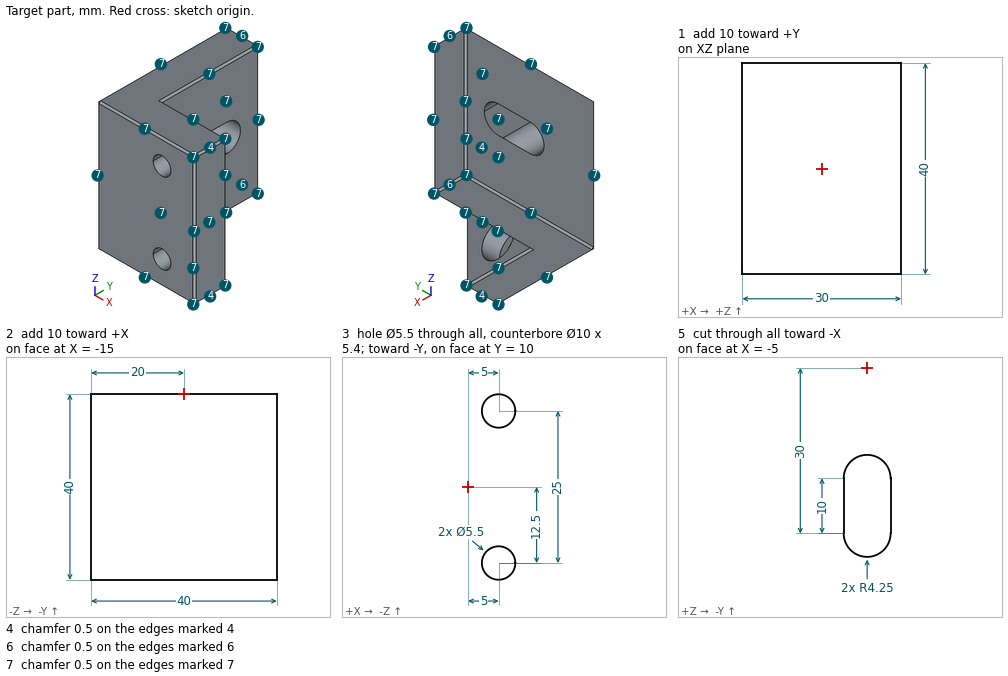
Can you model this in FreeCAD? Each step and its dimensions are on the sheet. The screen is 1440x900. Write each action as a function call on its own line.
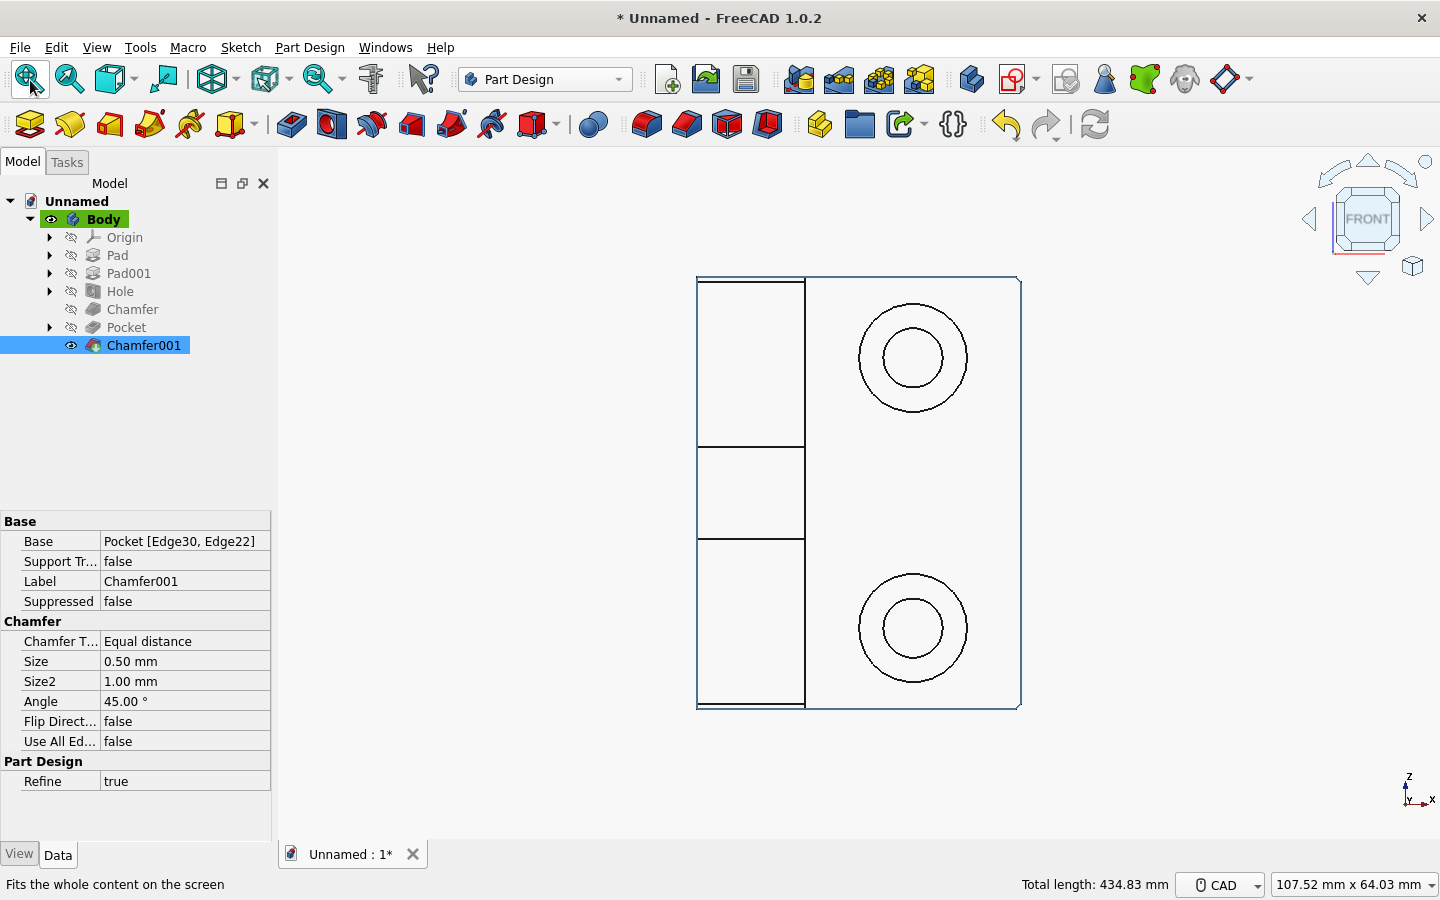
scroll(1018, 705, up, 9)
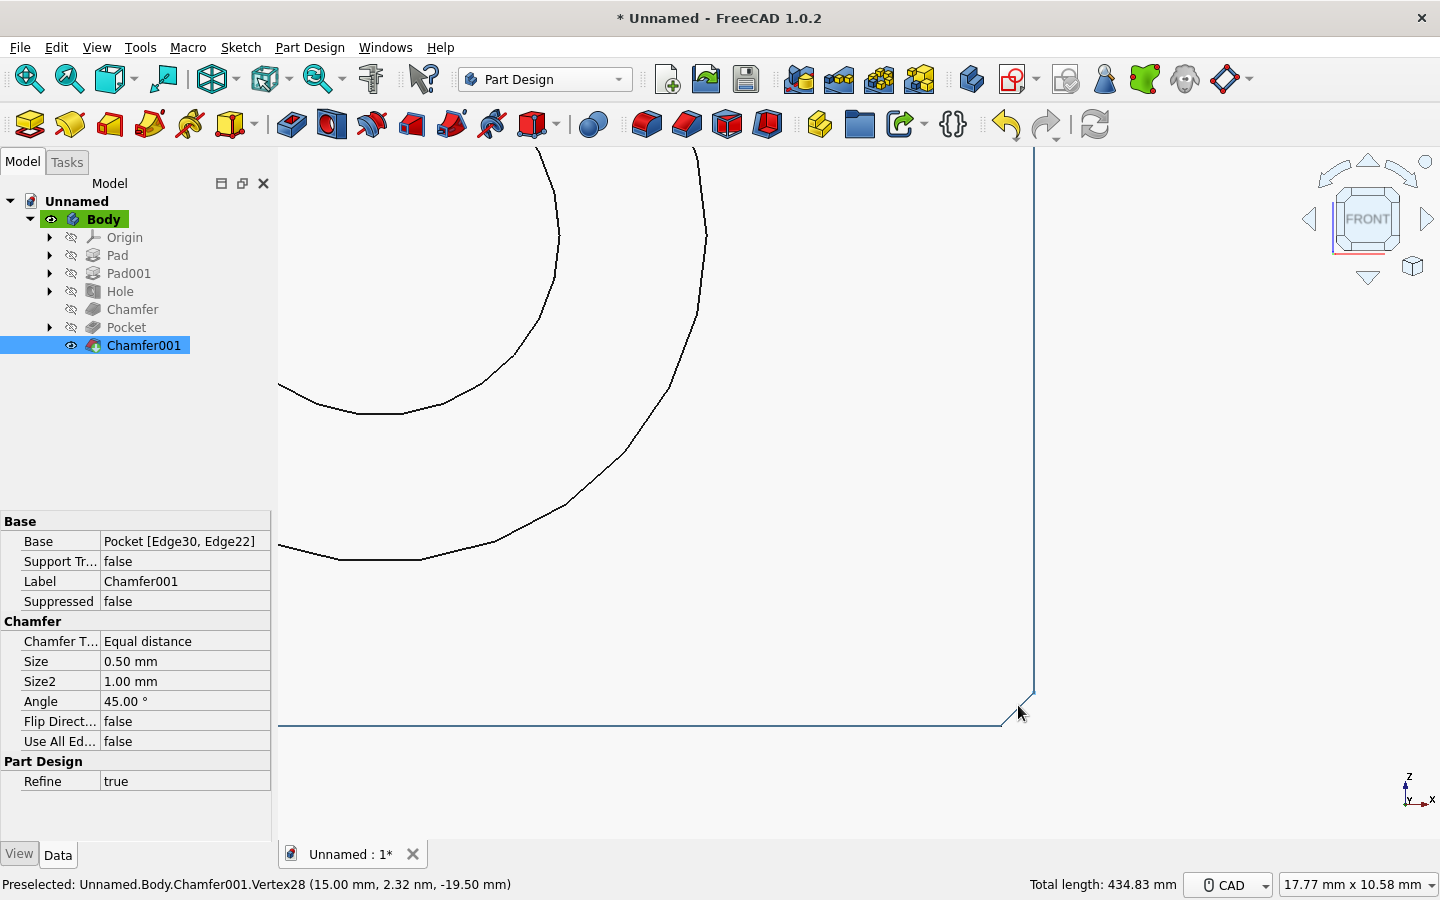
click(30, 80)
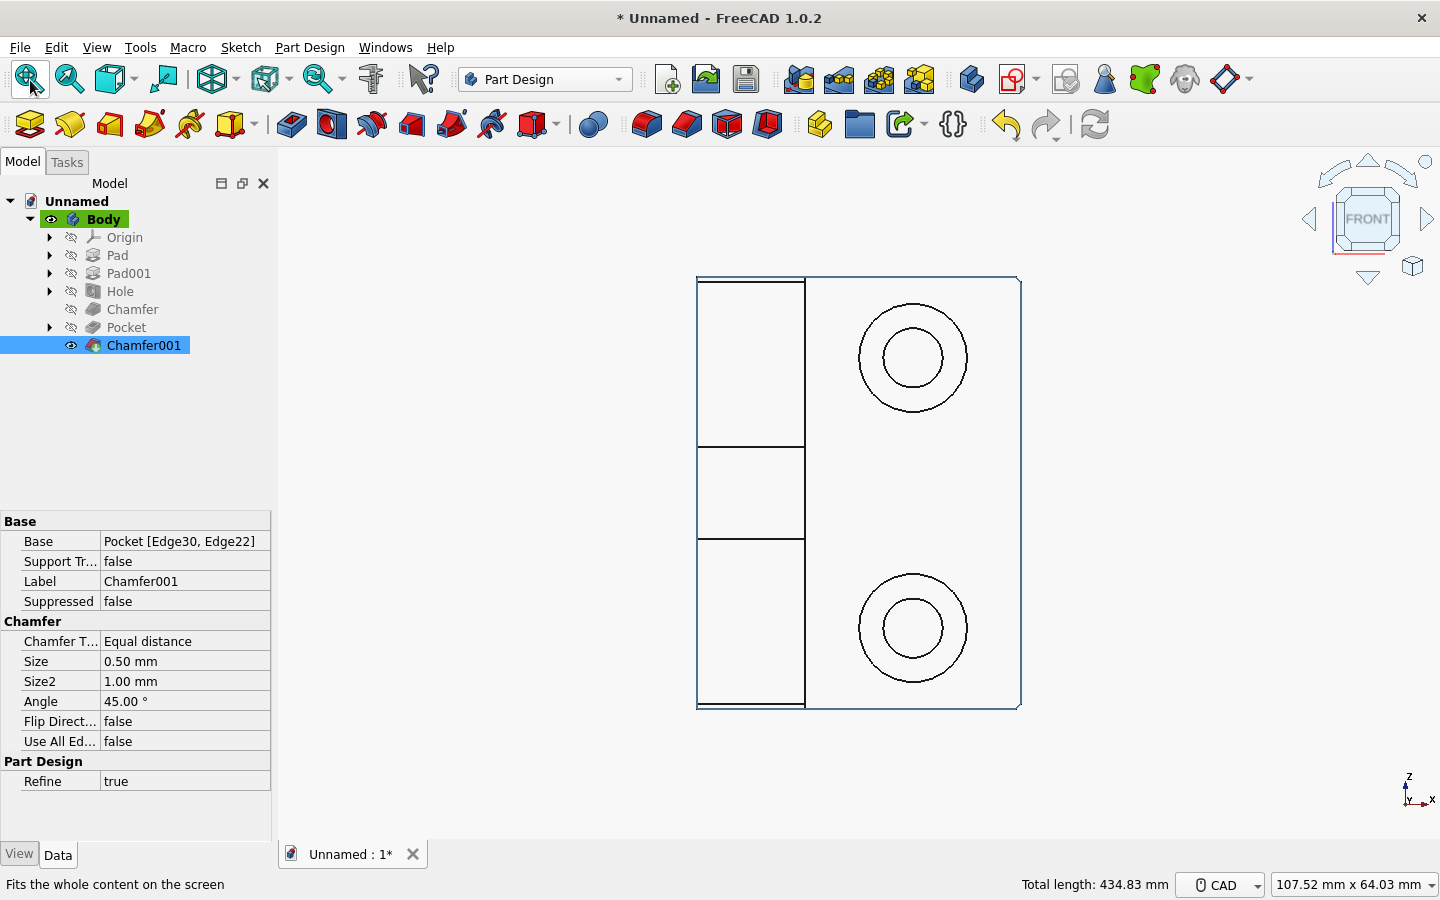
key(3)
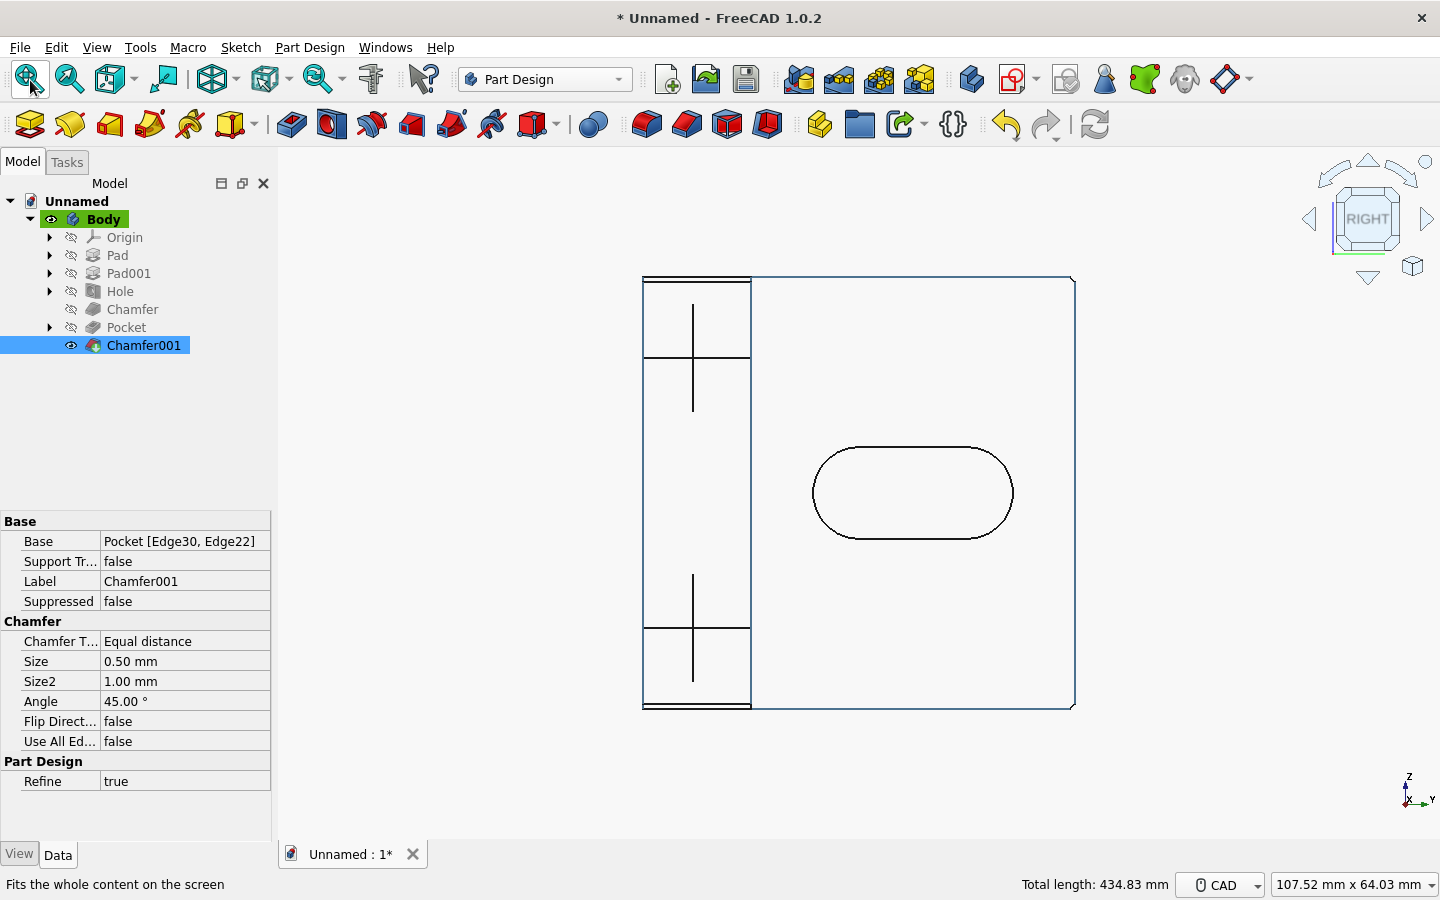
scroll(751, 705, up, 9)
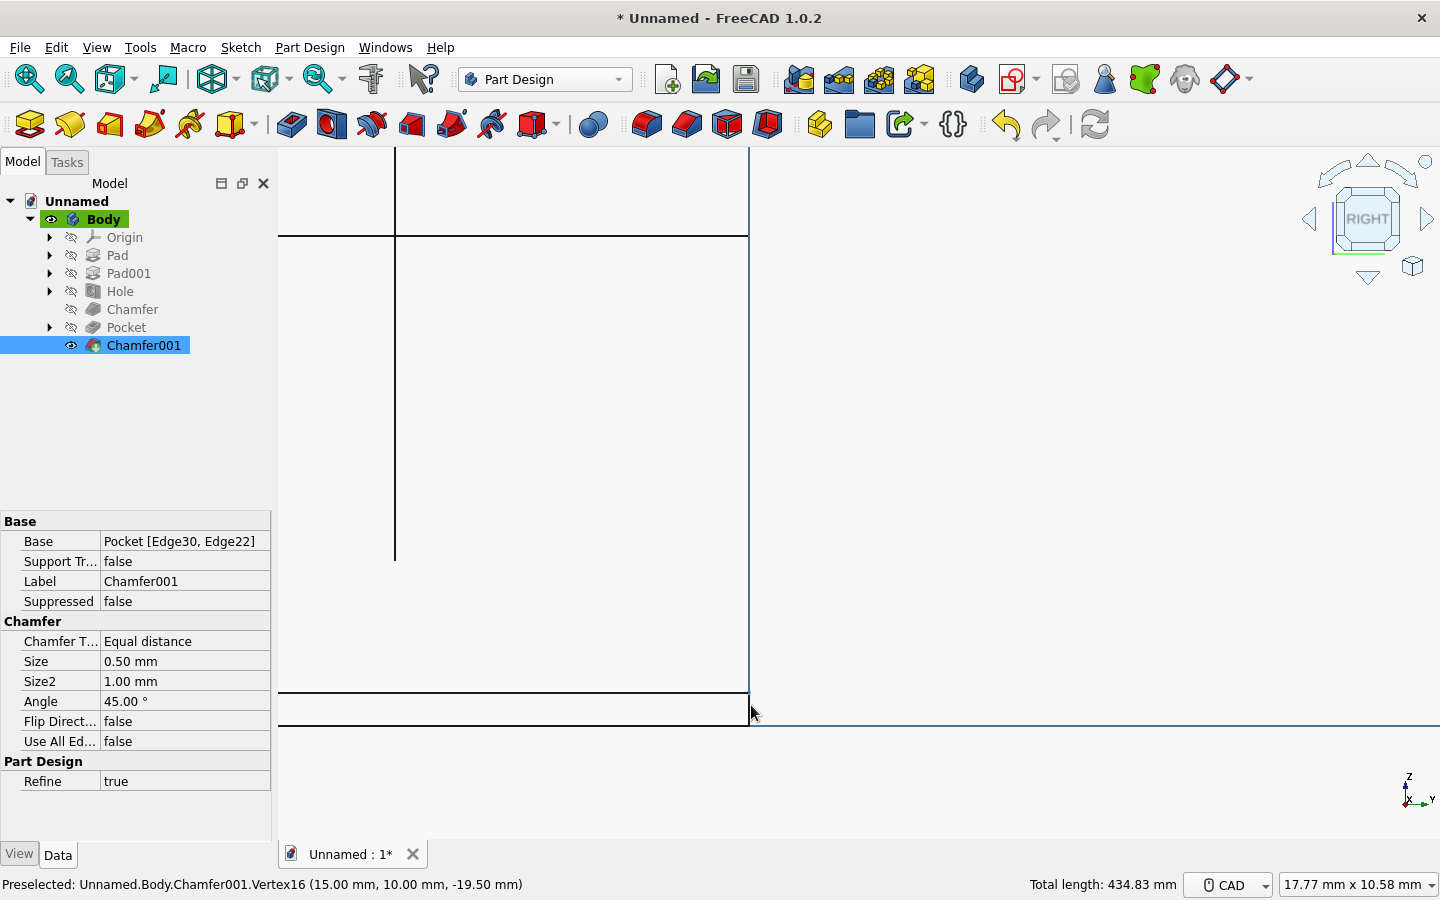
click(749, 709, ctrl)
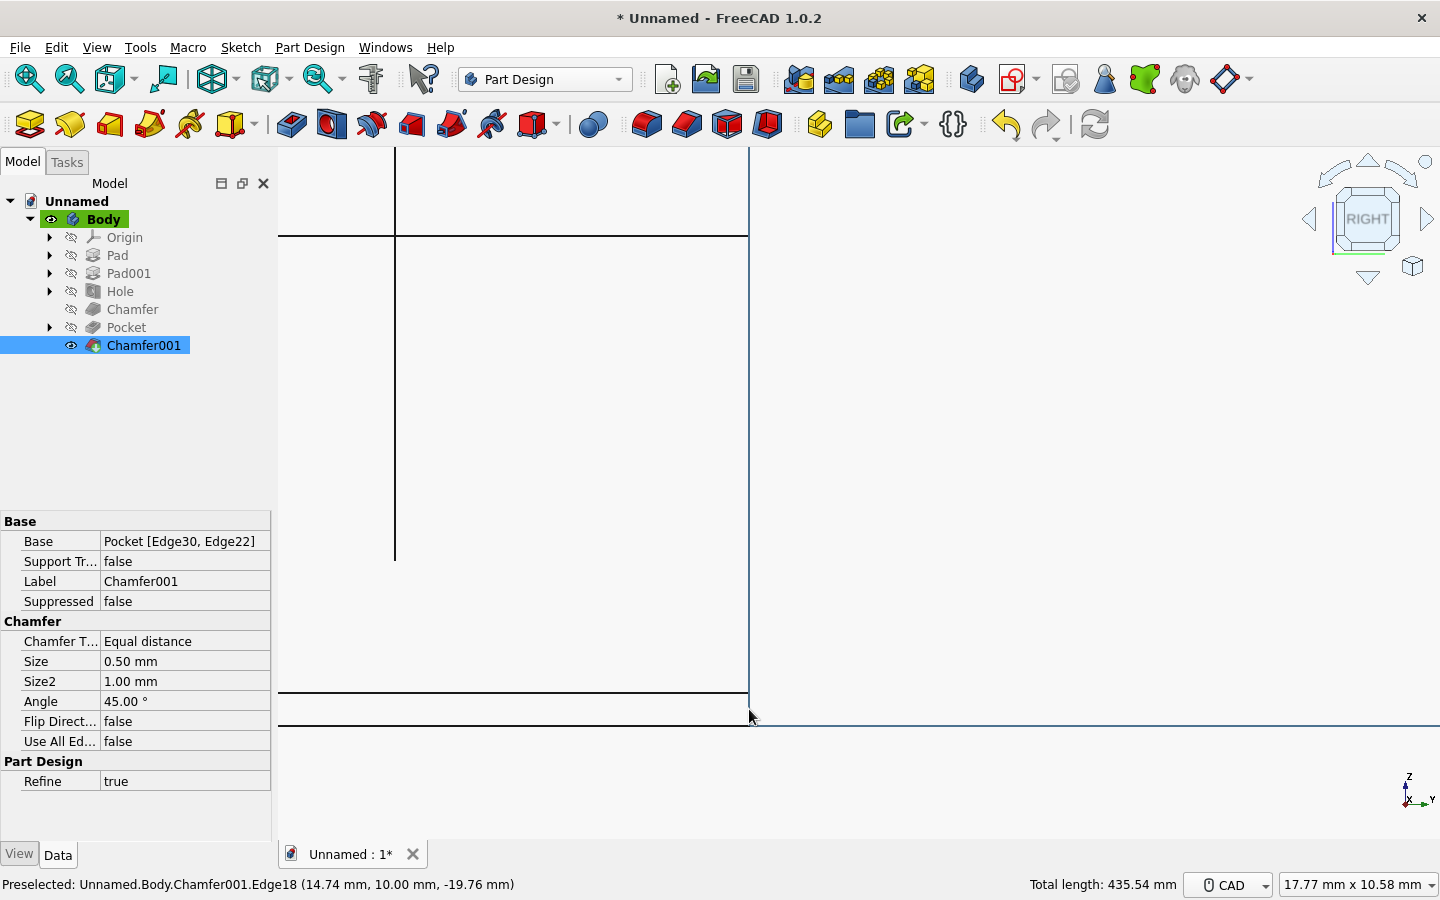
click(30, 80)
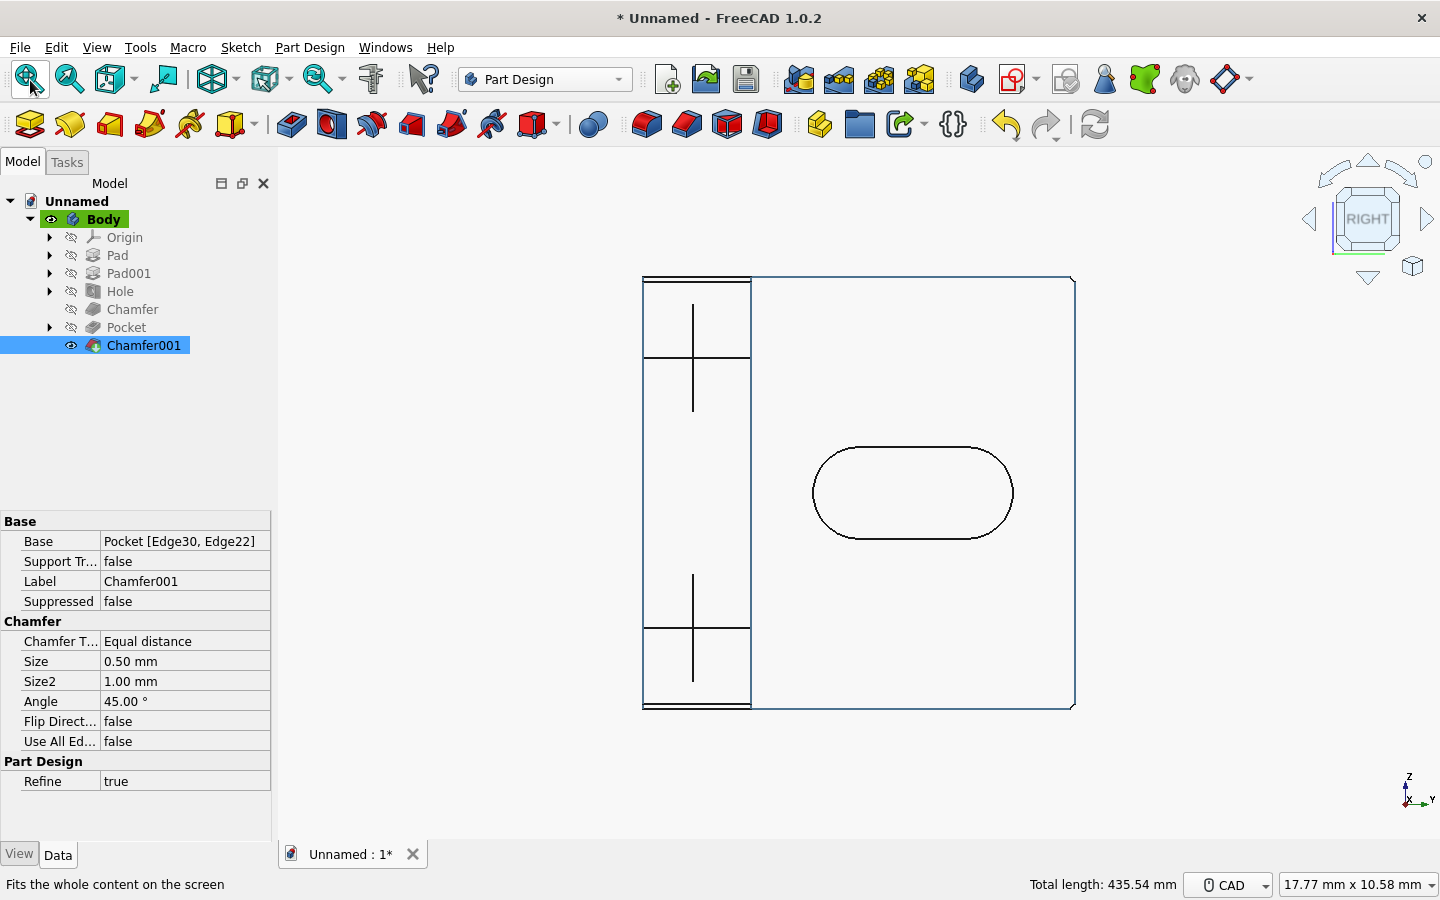
key(5)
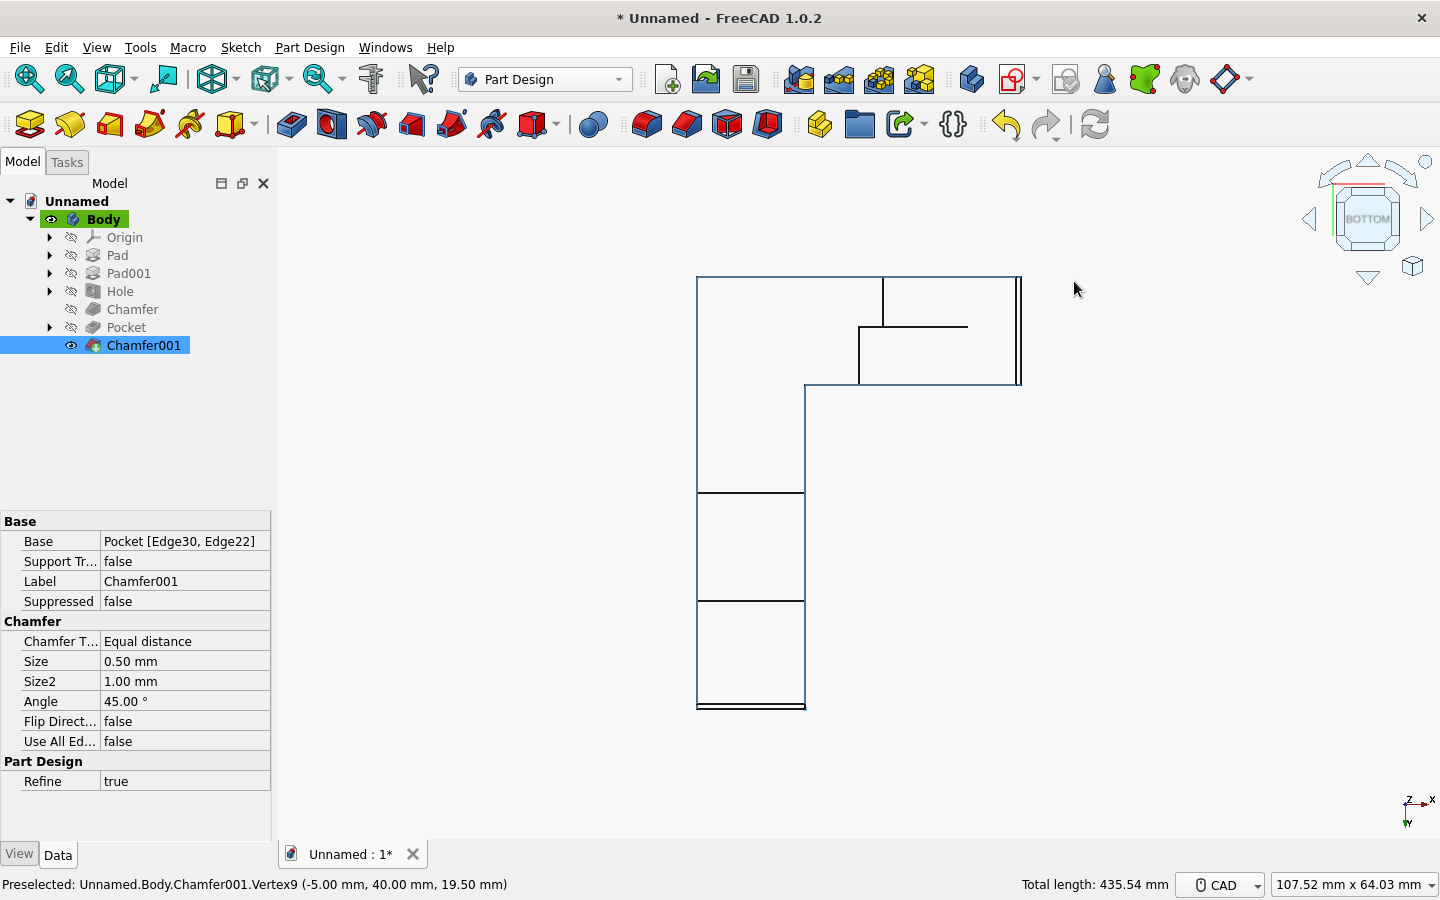
scroll(697, 705, up, 9)